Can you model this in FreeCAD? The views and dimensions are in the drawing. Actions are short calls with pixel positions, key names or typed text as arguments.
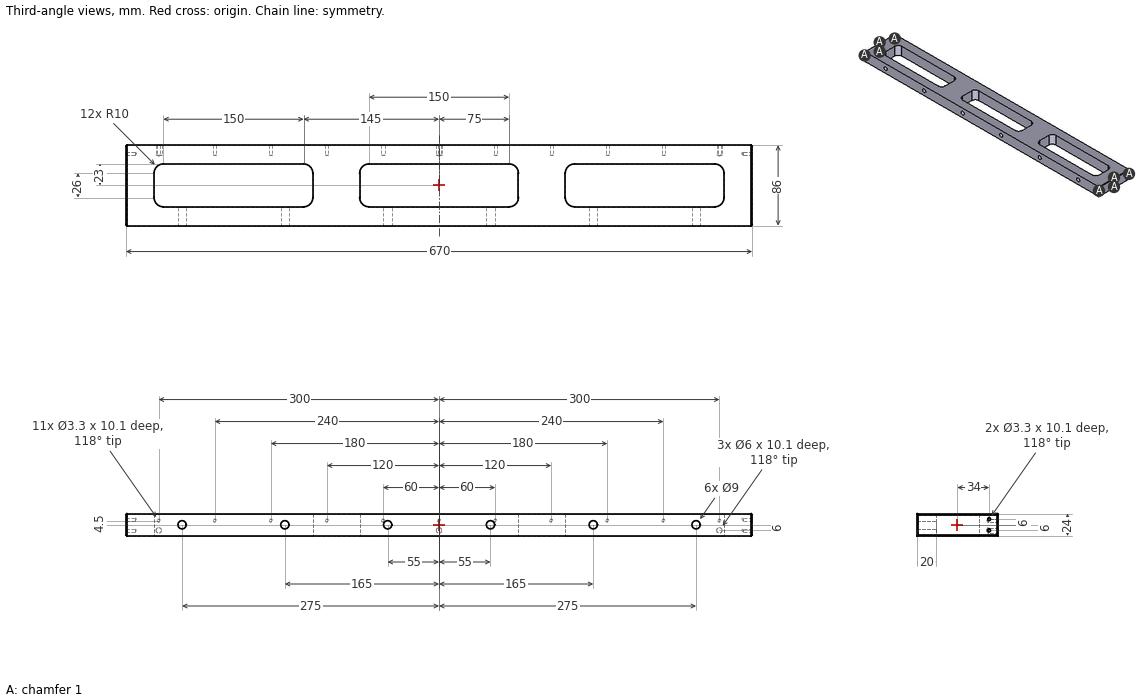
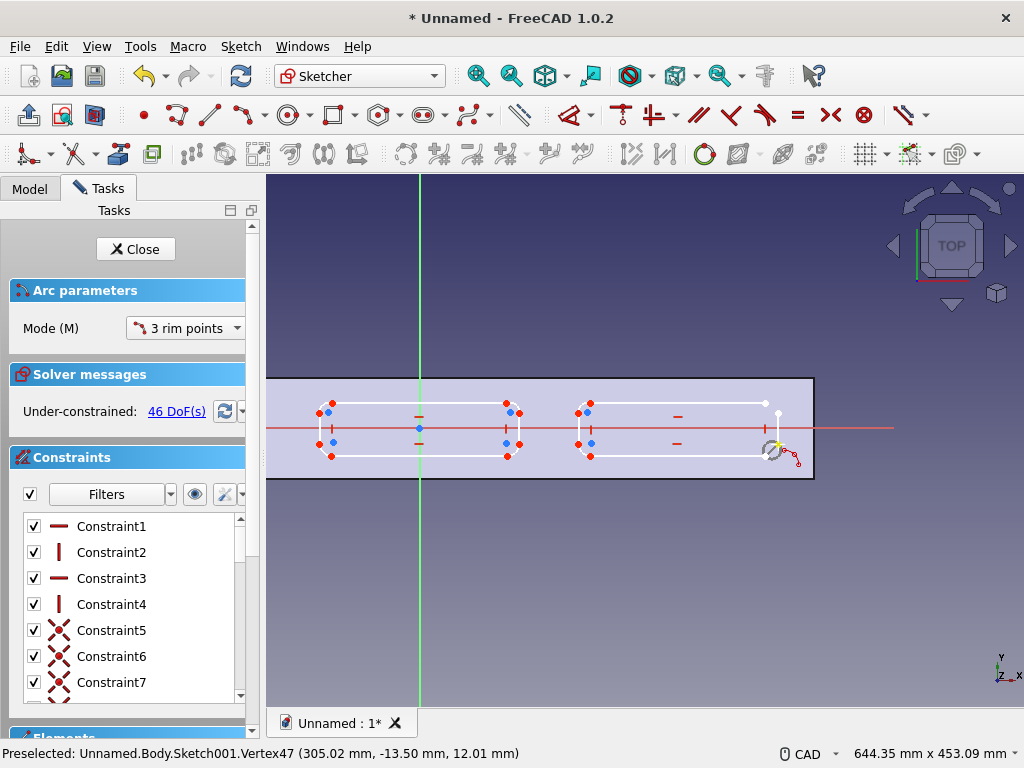
scroll(775, 452, up, 8)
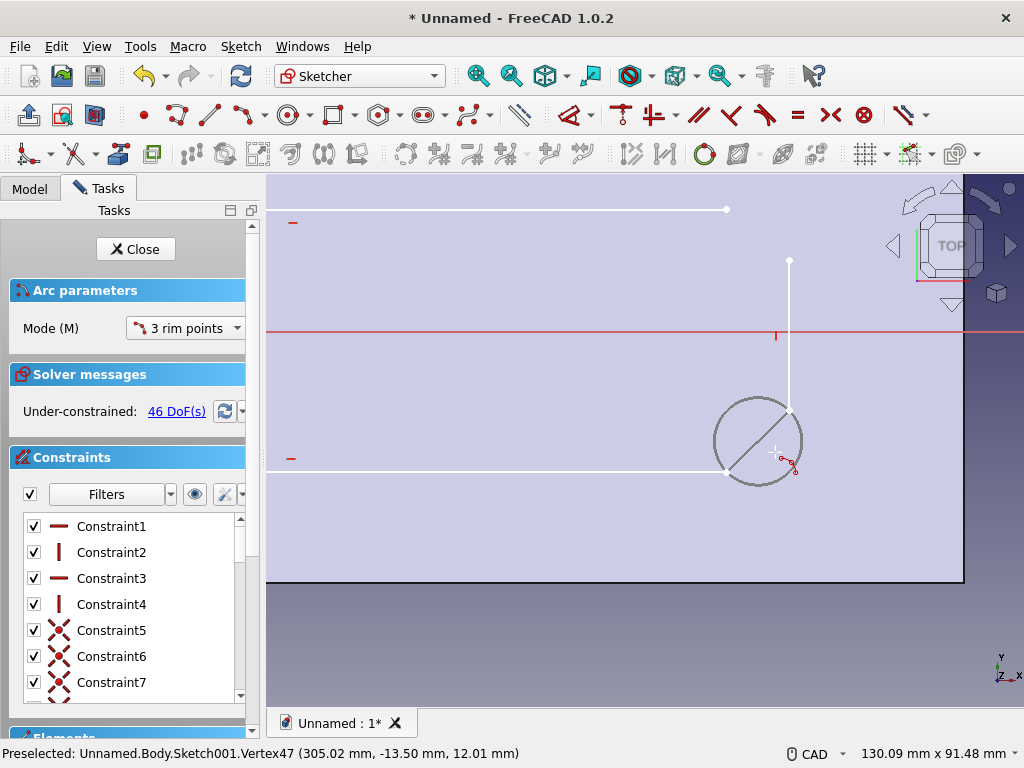
click(772, 449)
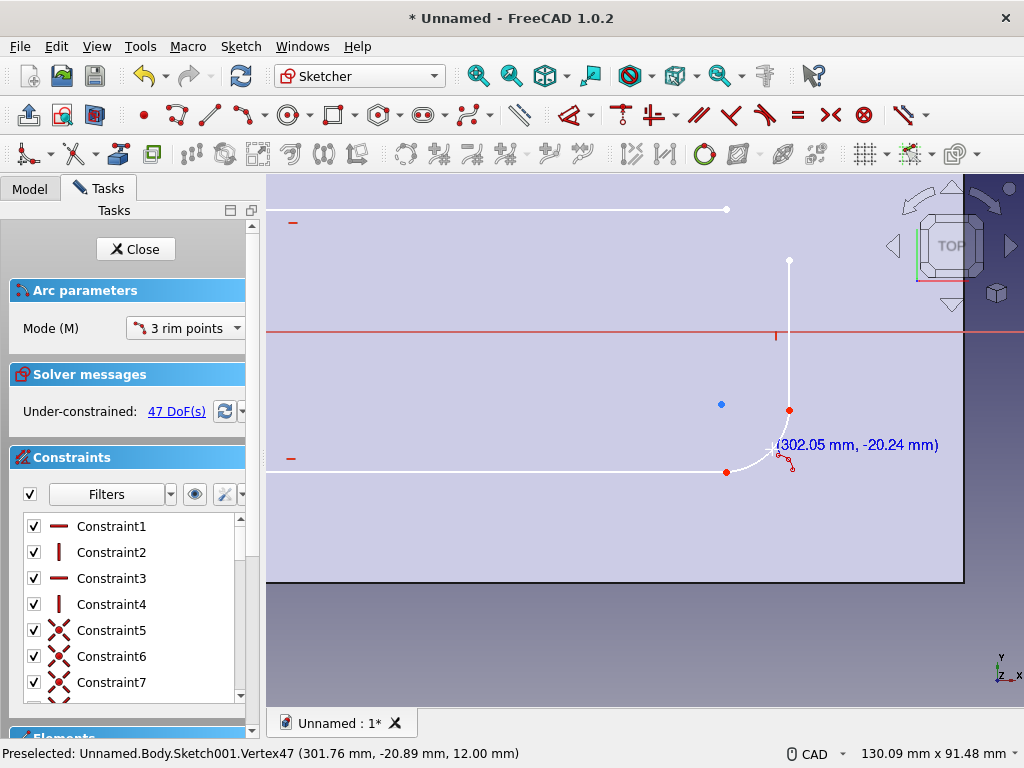
scroll(771, 454, down, 11)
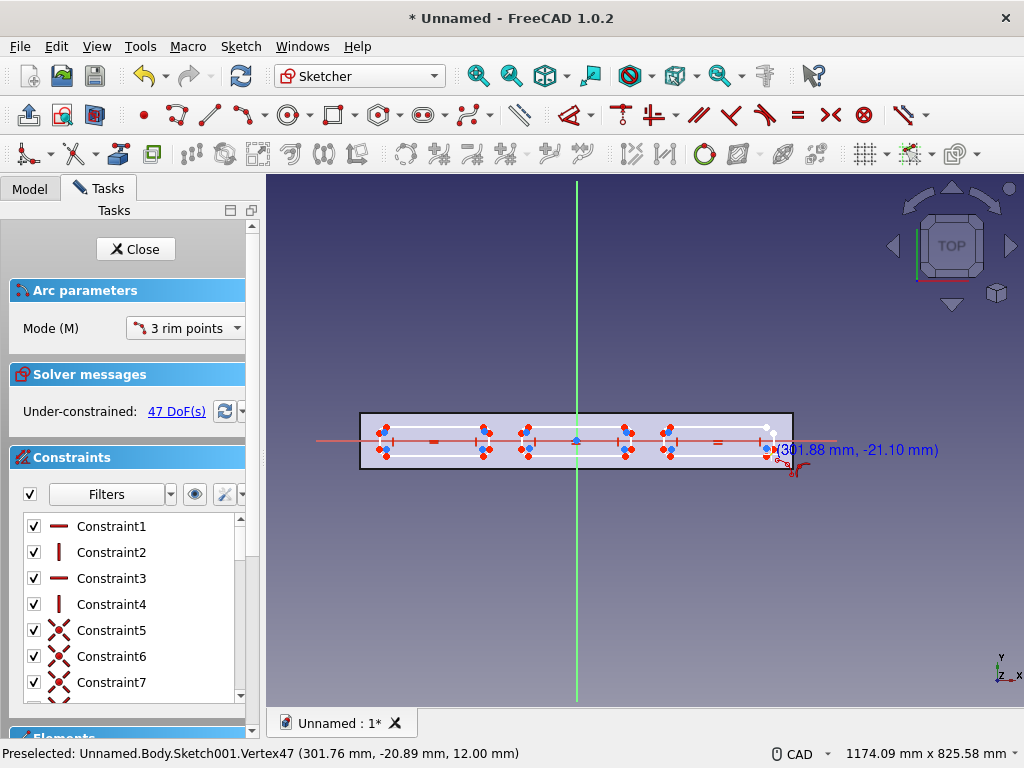
scroll(774, 433, up, 4)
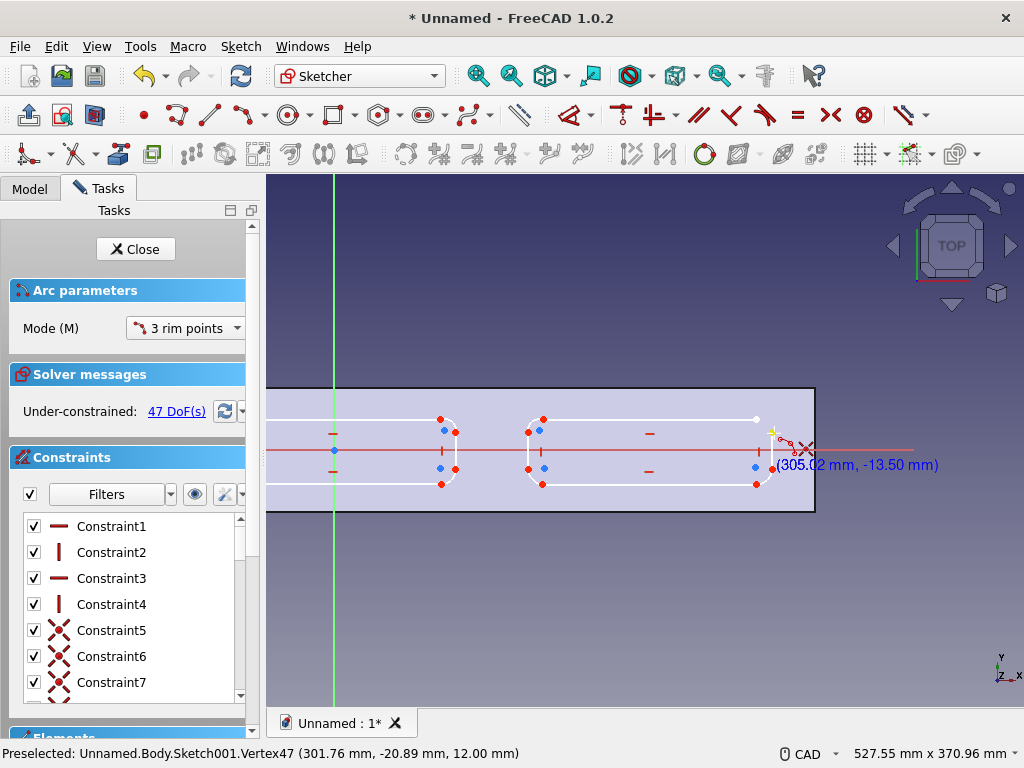
click(772, 433)
click(757, 420)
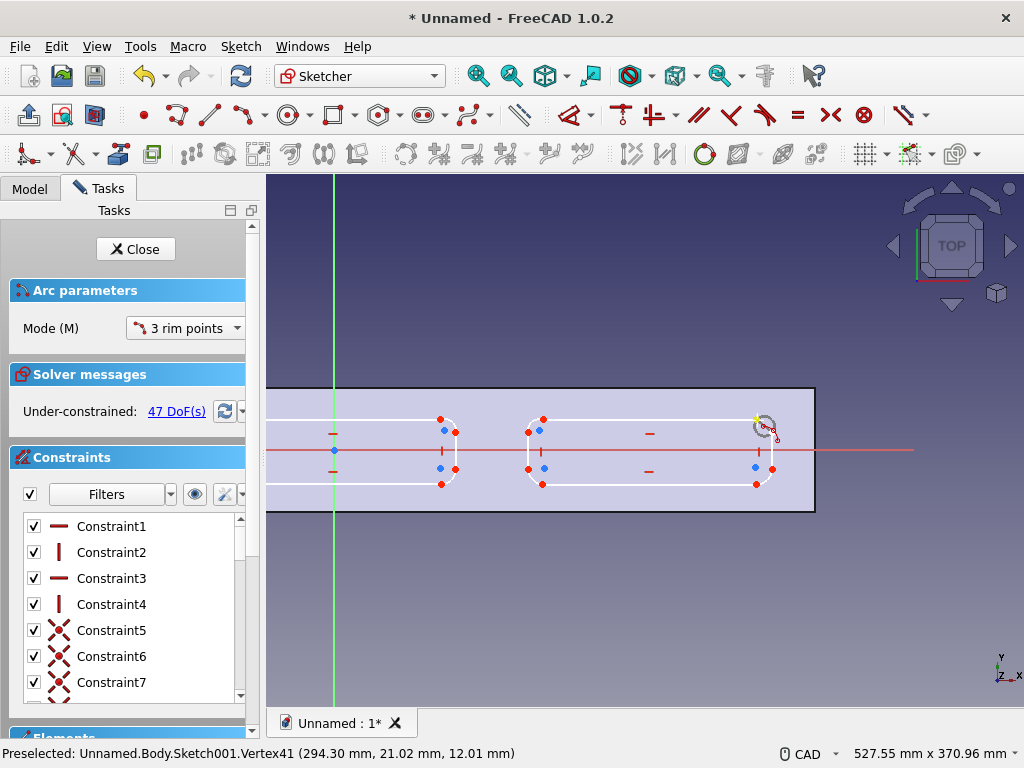
scroll(768, 421, up, 7)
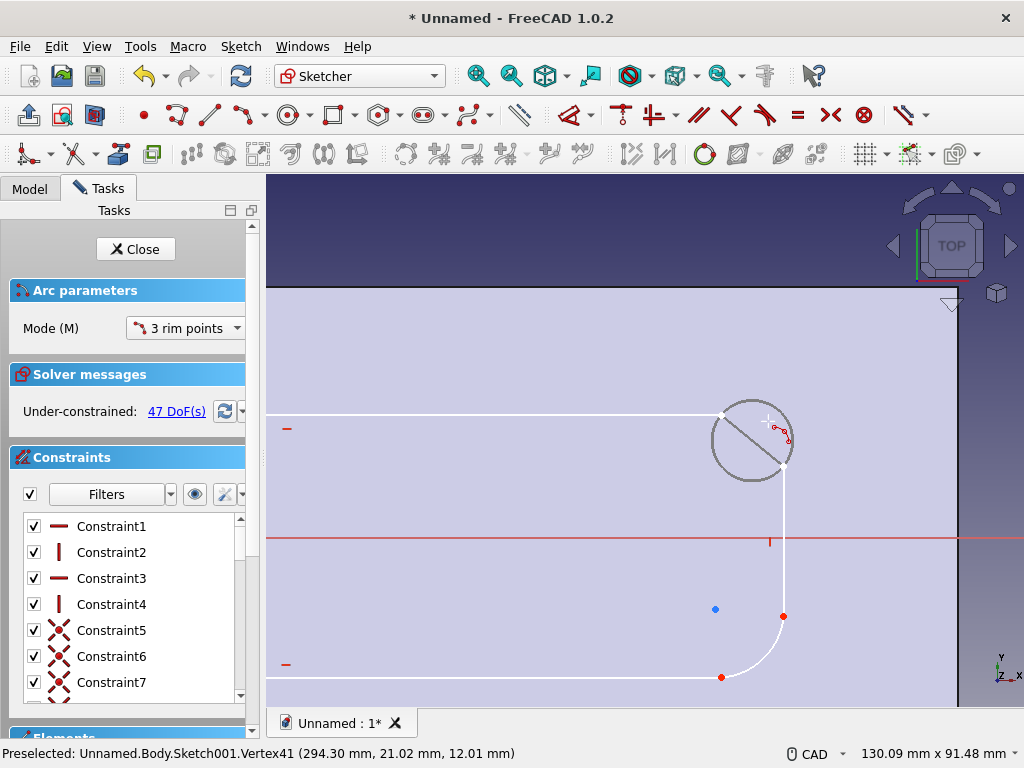
click(766, 421)
key(Escape)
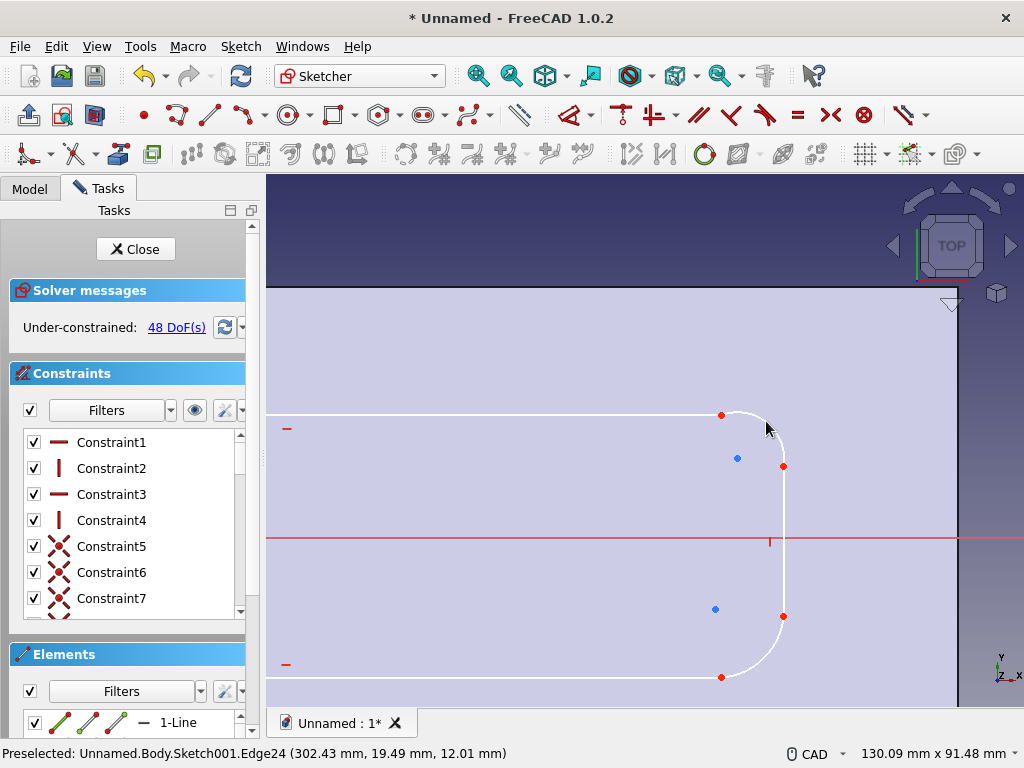
scroll(772, 428, down, 11)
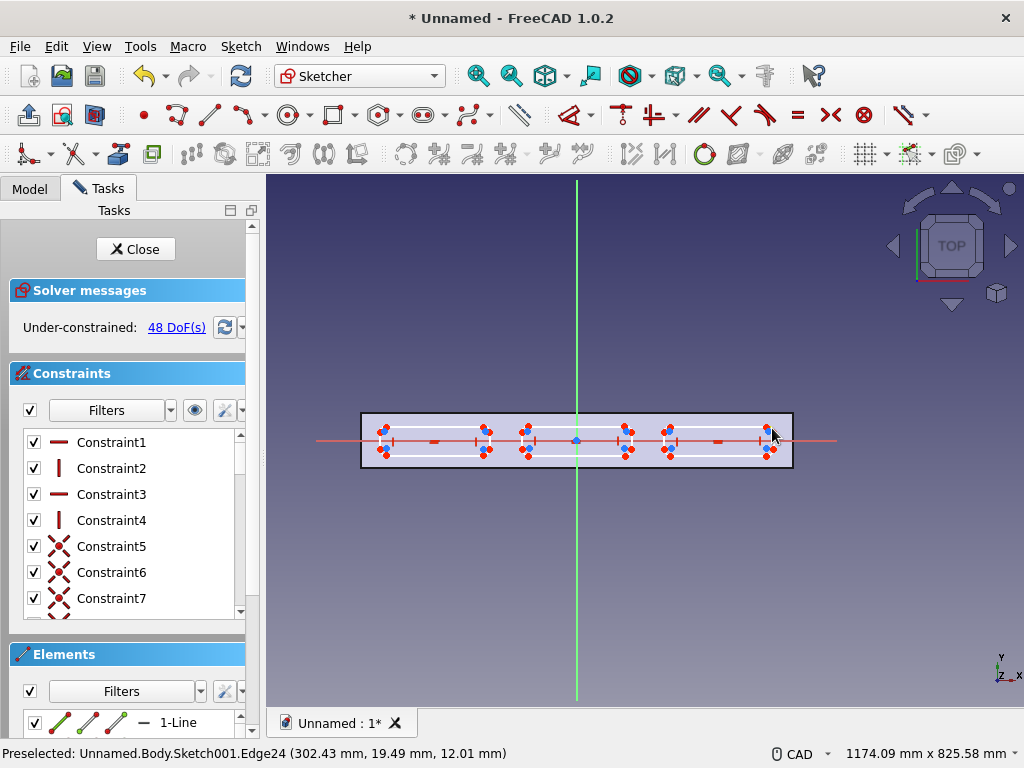
click(454, 427)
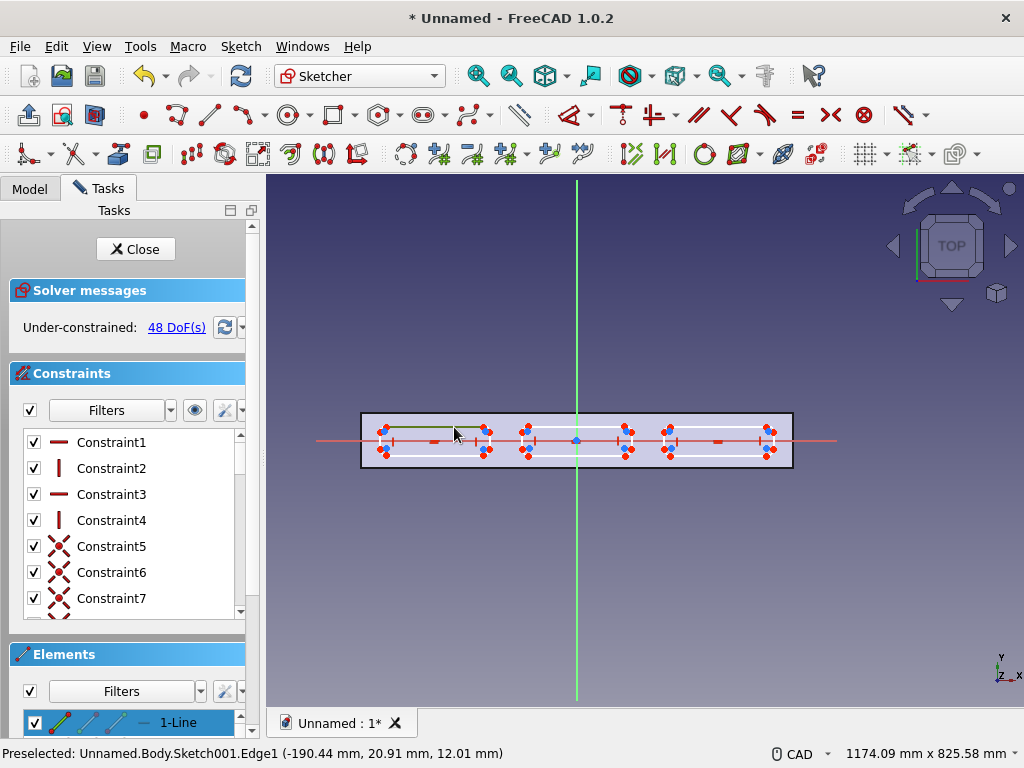
scroll(382, 428, up, 6)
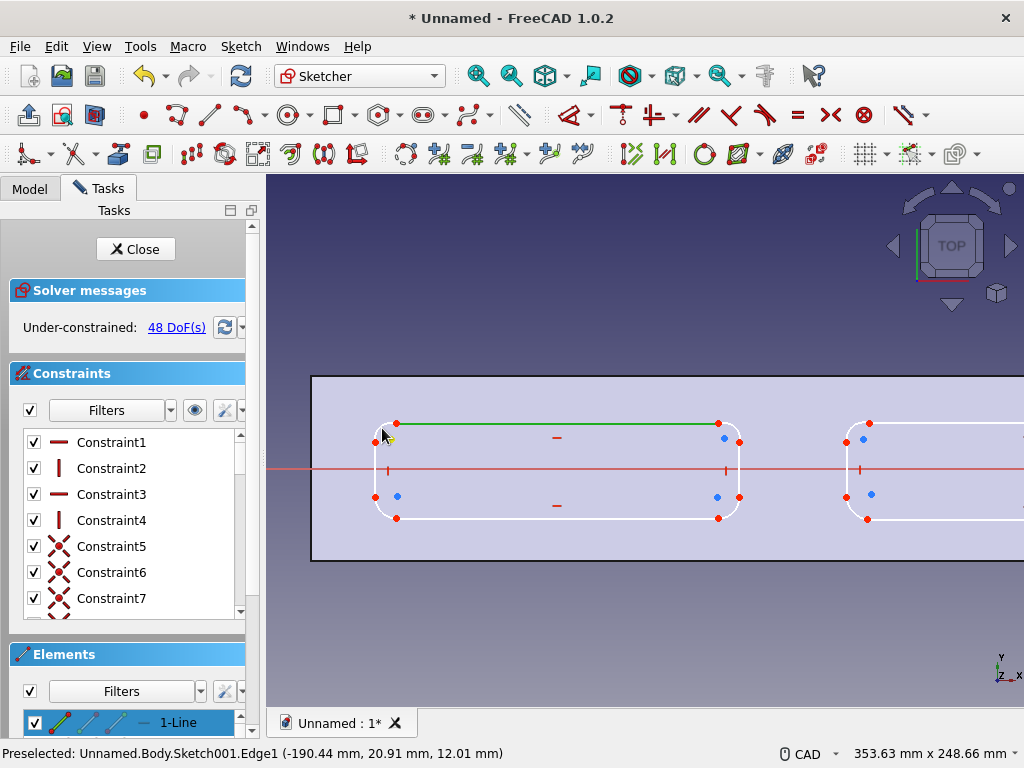
click(380, 427)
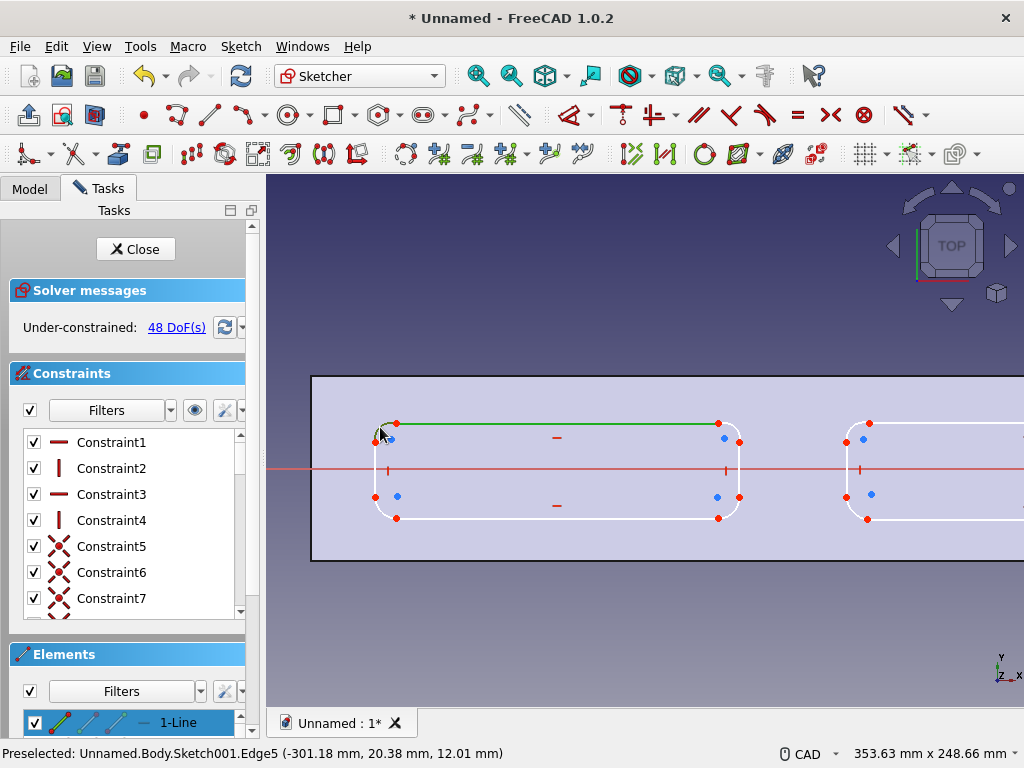
click(765, 116)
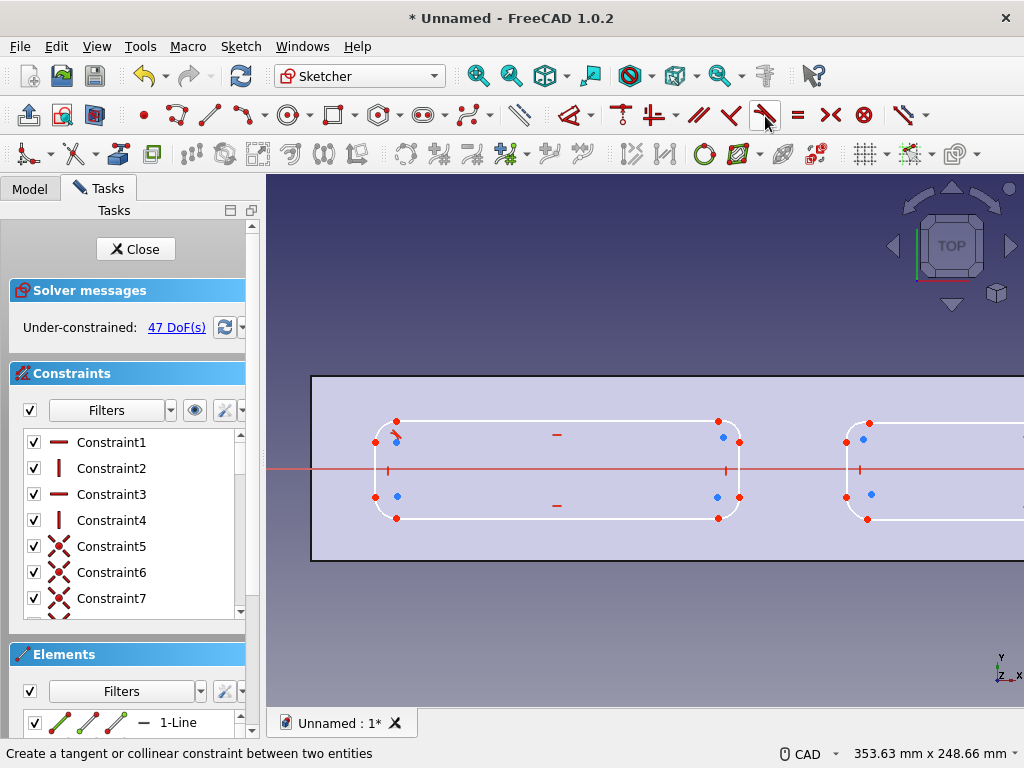
click(622, 421)